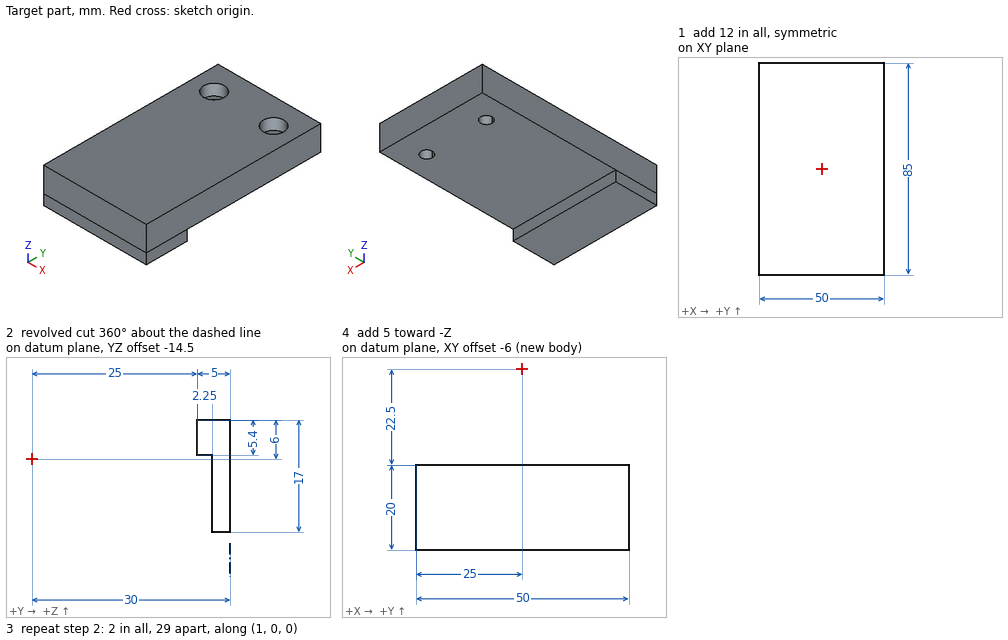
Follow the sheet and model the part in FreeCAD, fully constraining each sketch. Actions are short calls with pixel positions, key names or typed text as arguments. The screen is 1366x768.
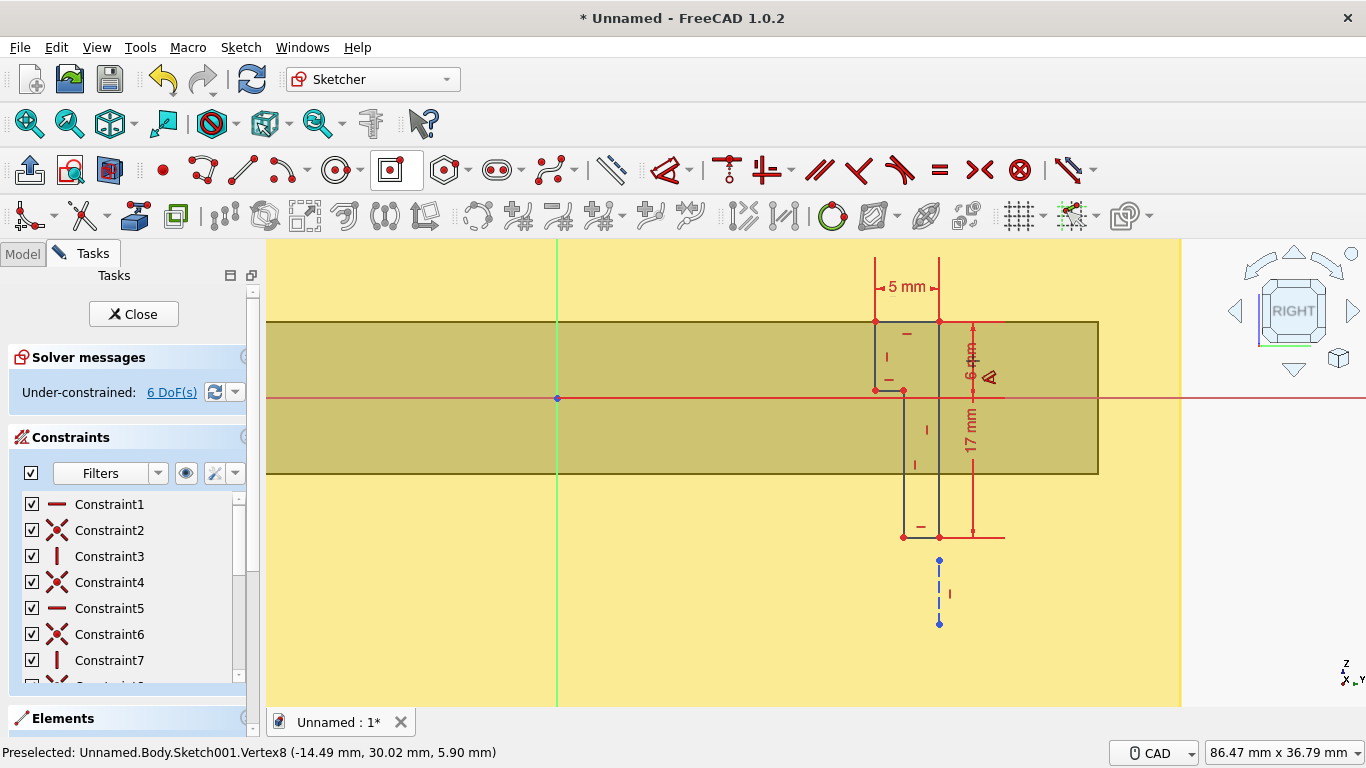
click(875, 342)
click(909, 340)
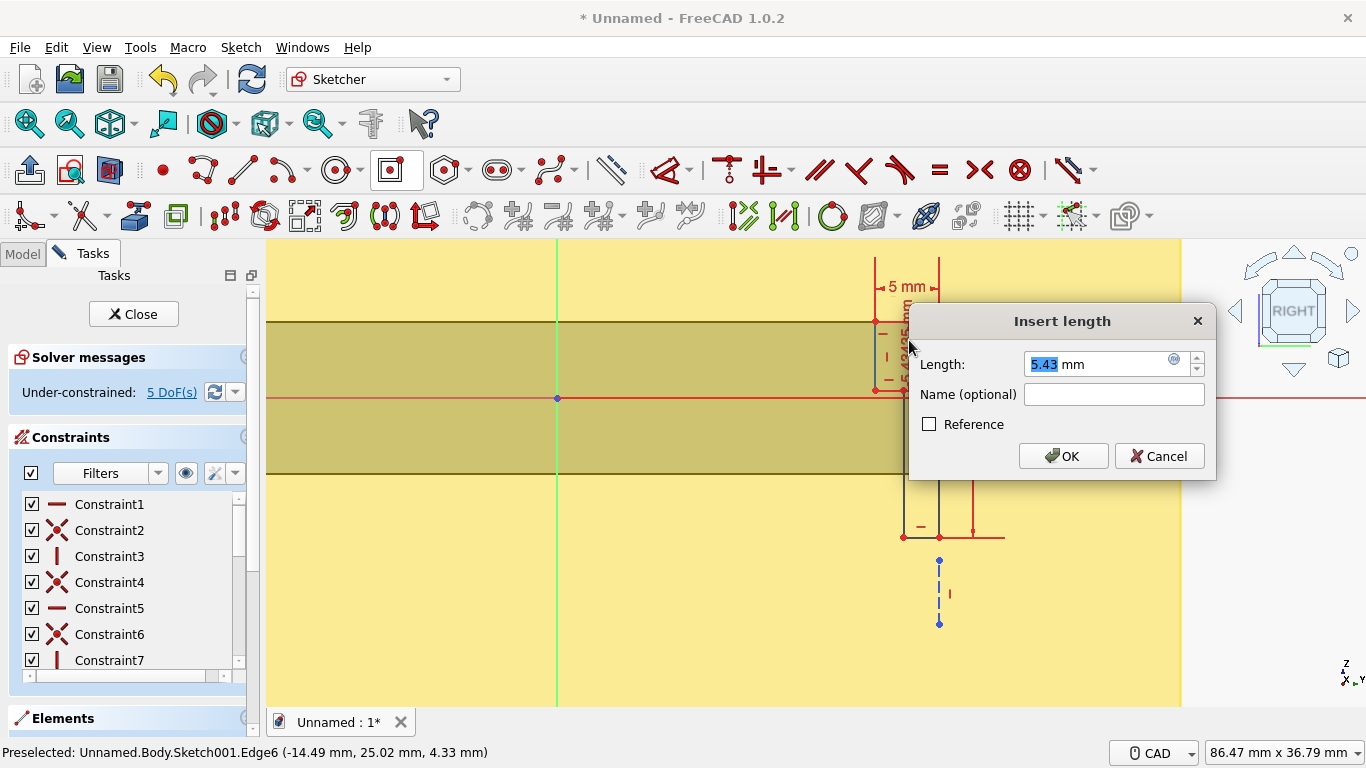
text(5.4)
key(Return)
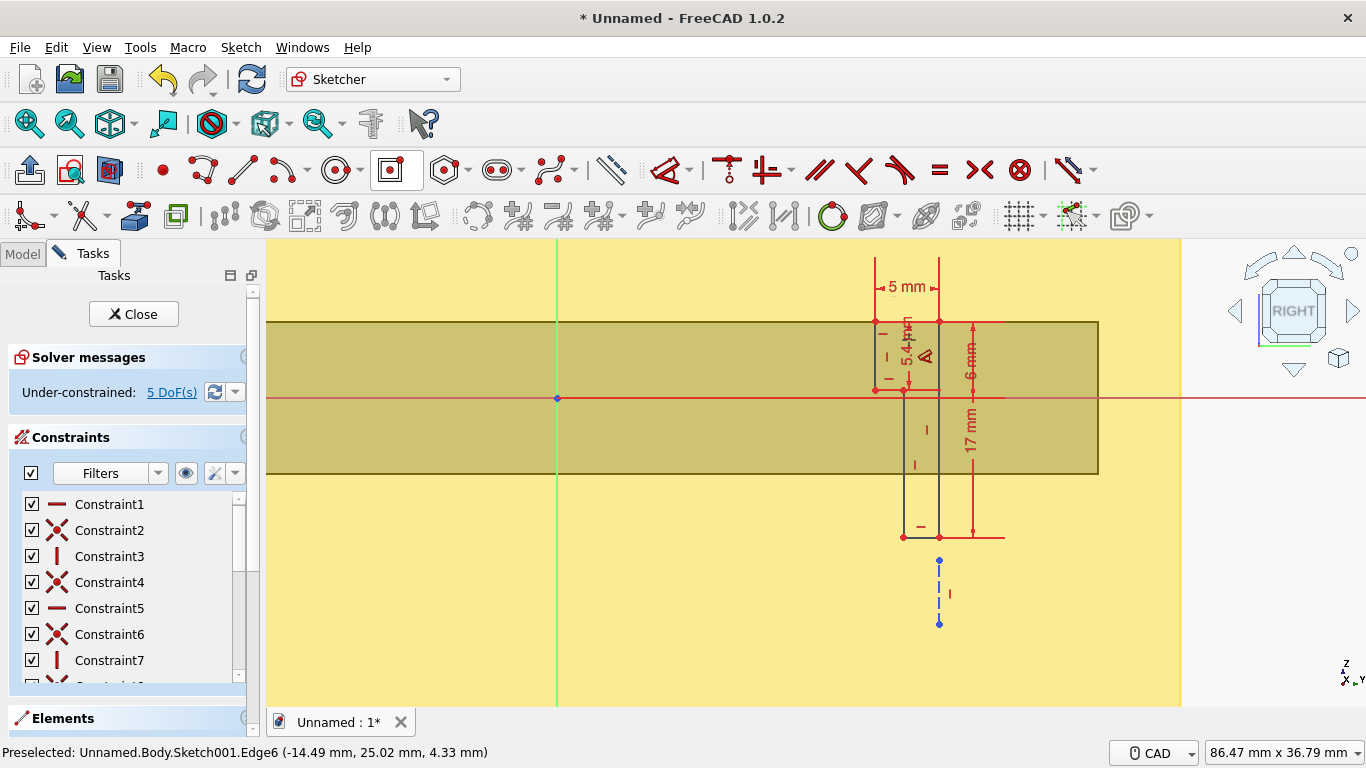
click(875, 390)
click(716, 356)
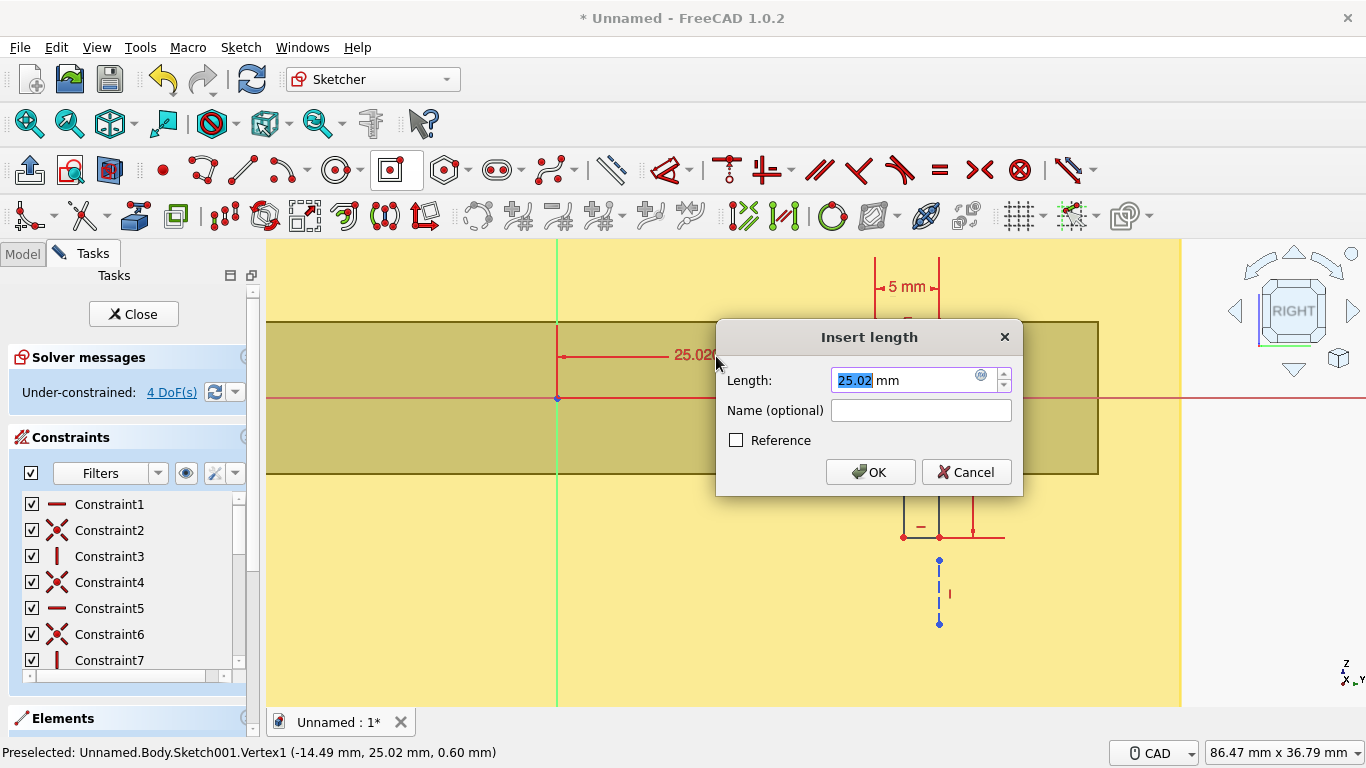
text(25)
key(Return)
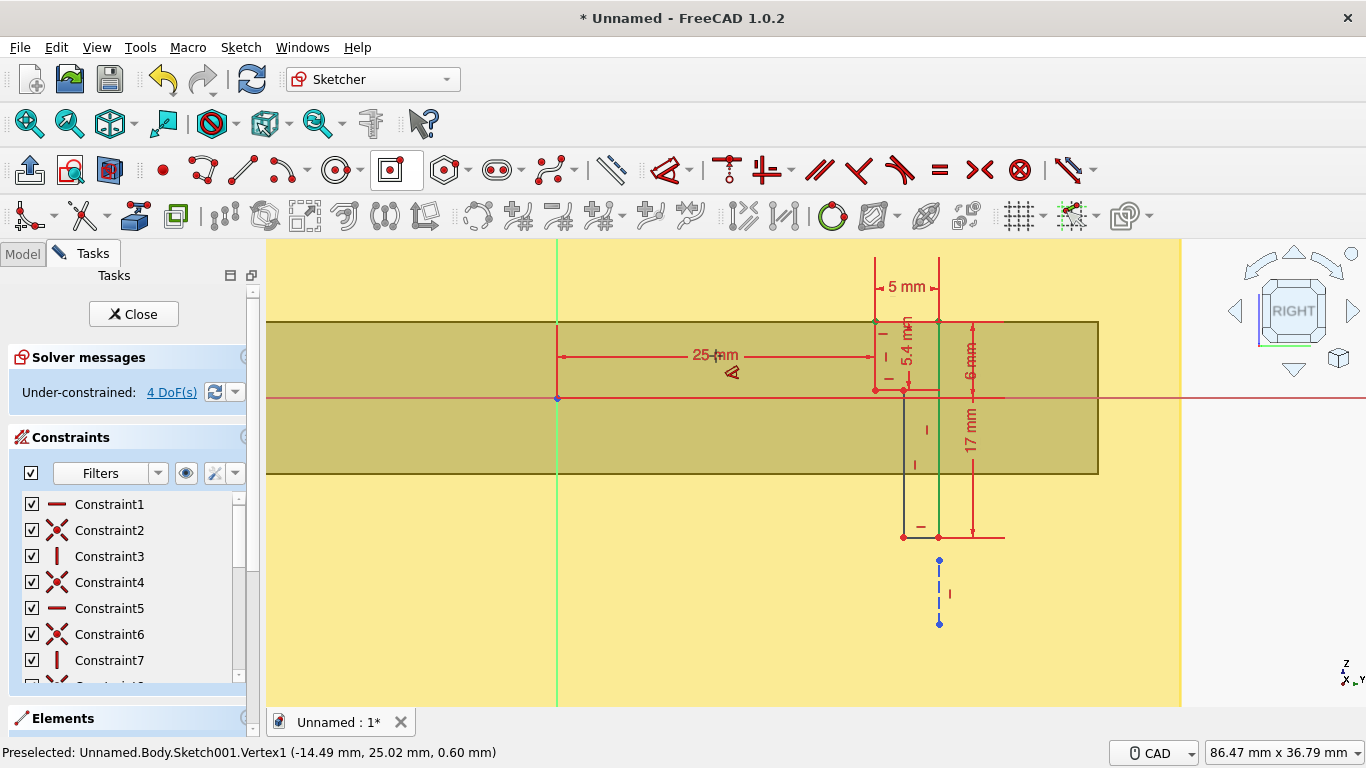
click(939, 561)
click(748, 595)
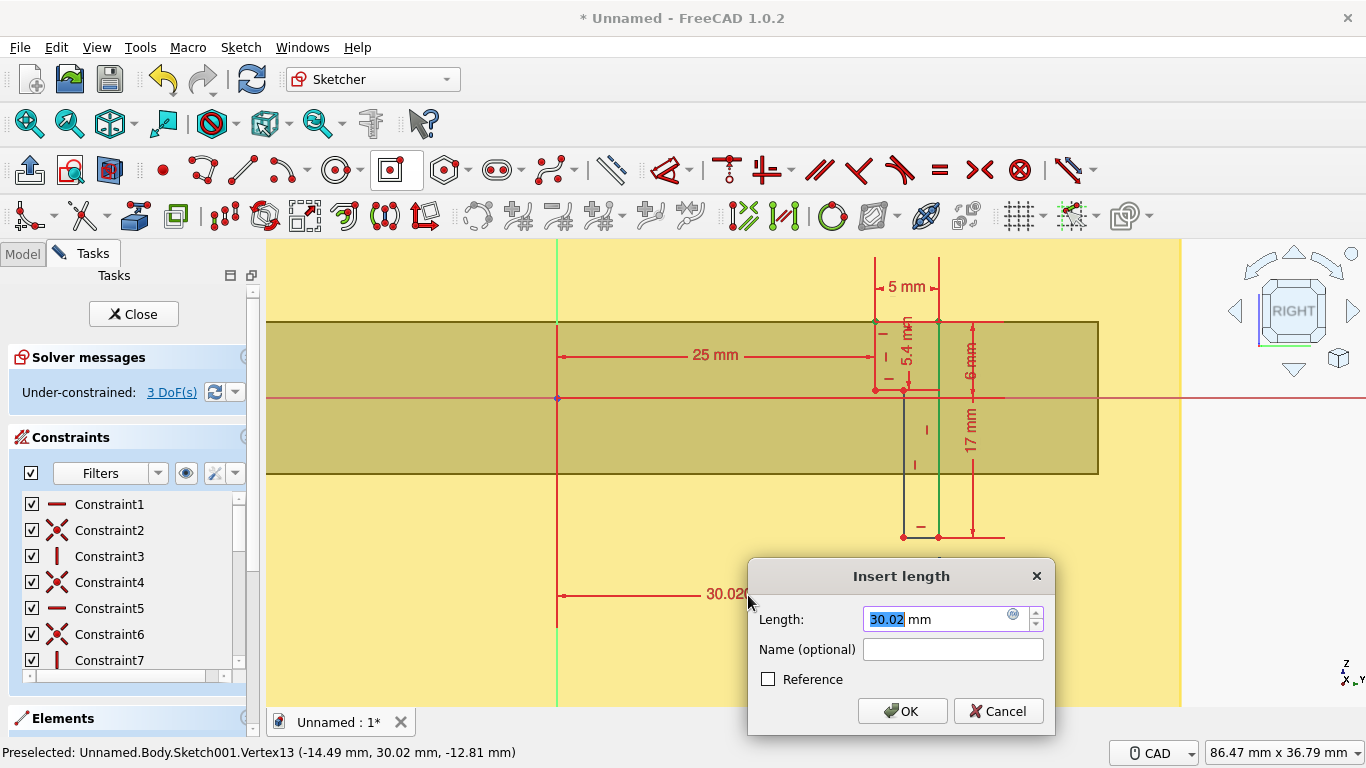
text(30)
key(Return)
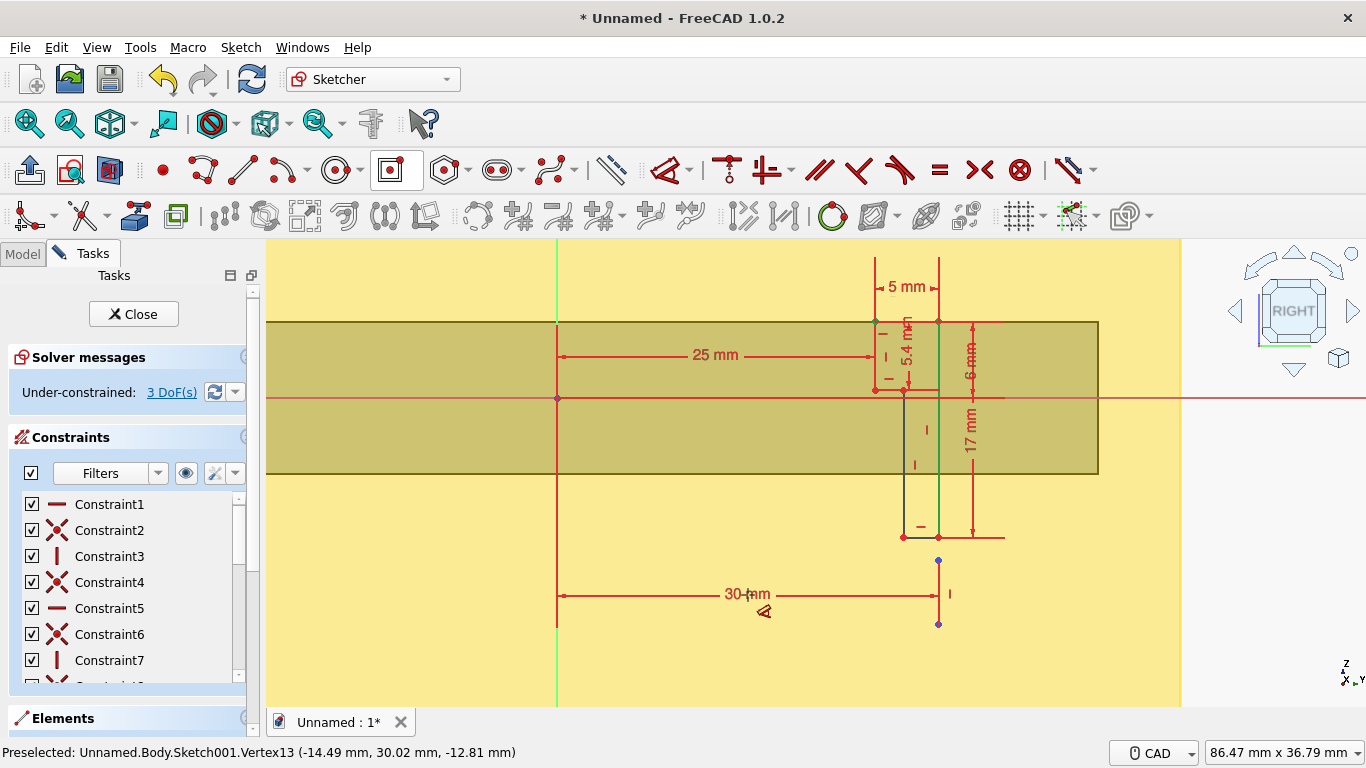
scroll(884, 390, up, 3)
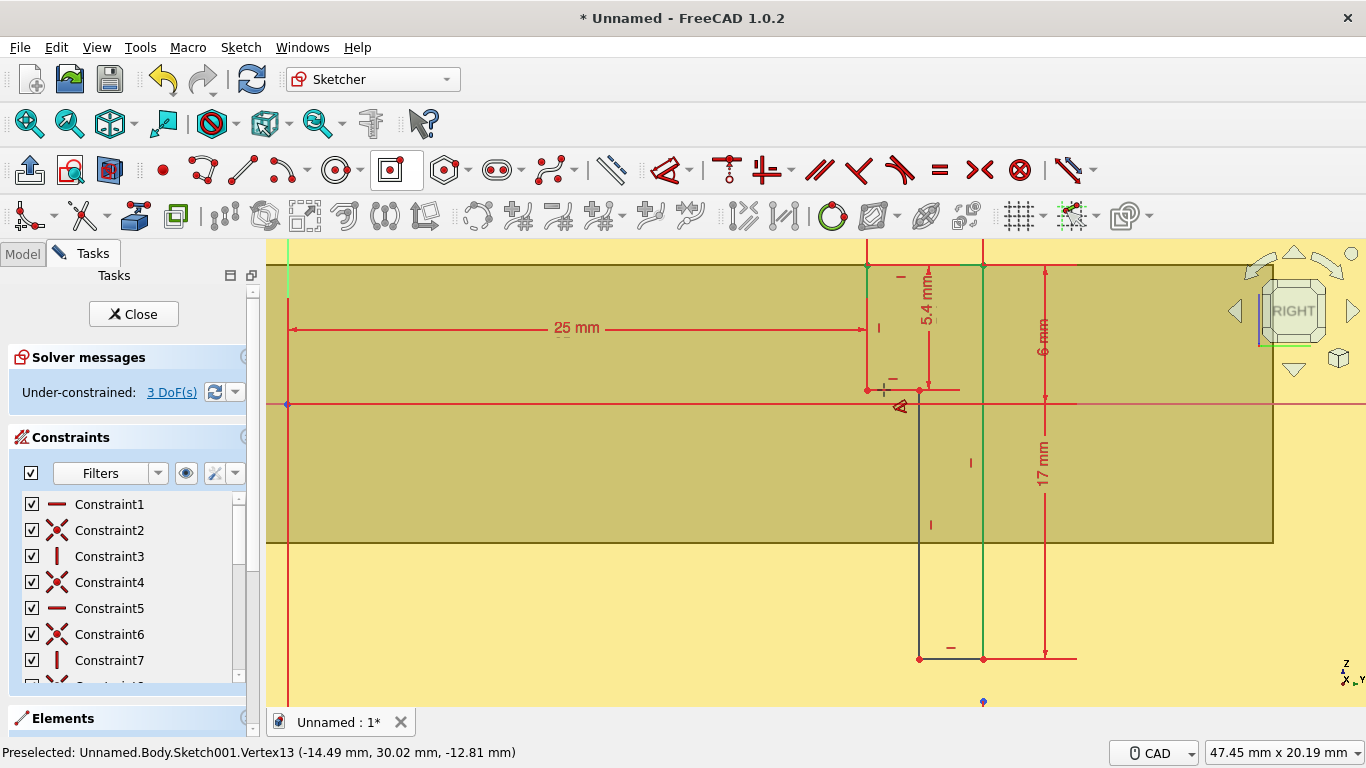
click(883, 390)
click(893, 356)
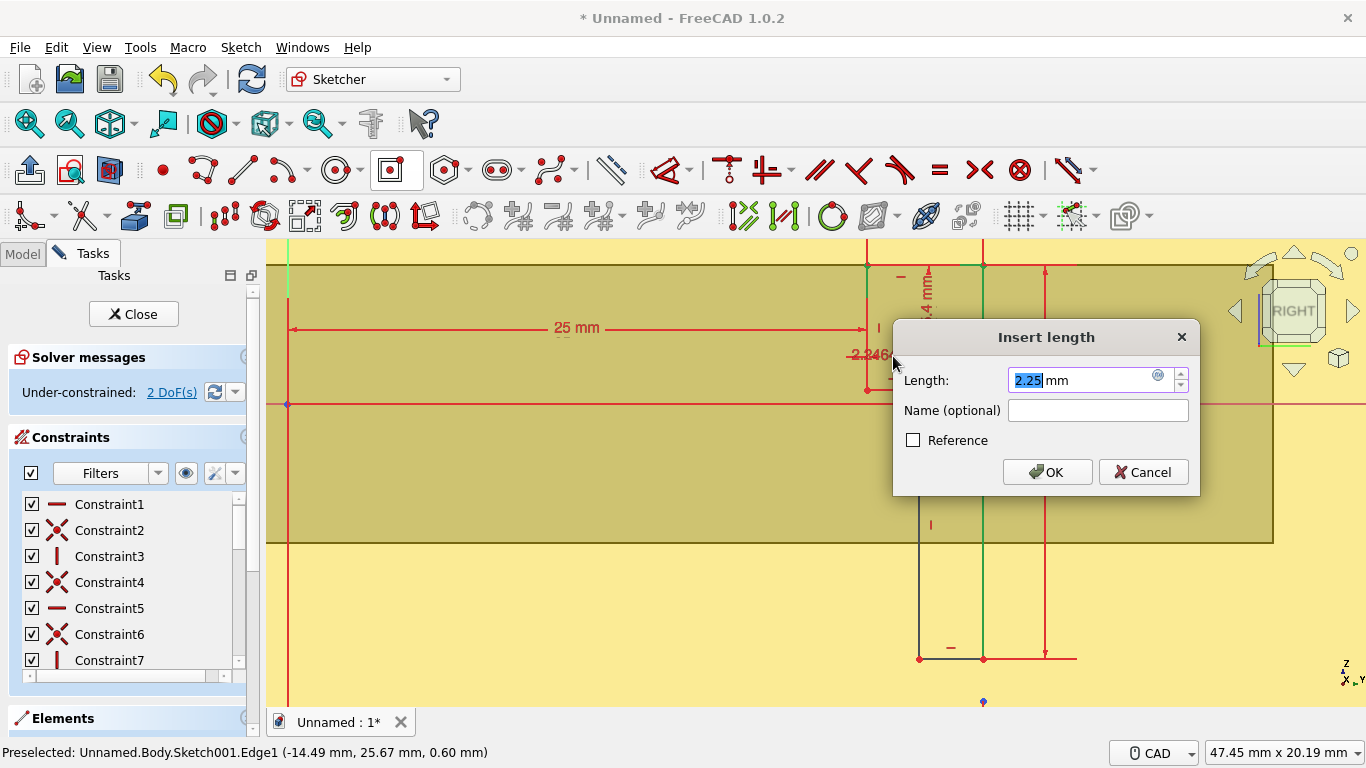
text(2.25)
key(Return)
key(Escape)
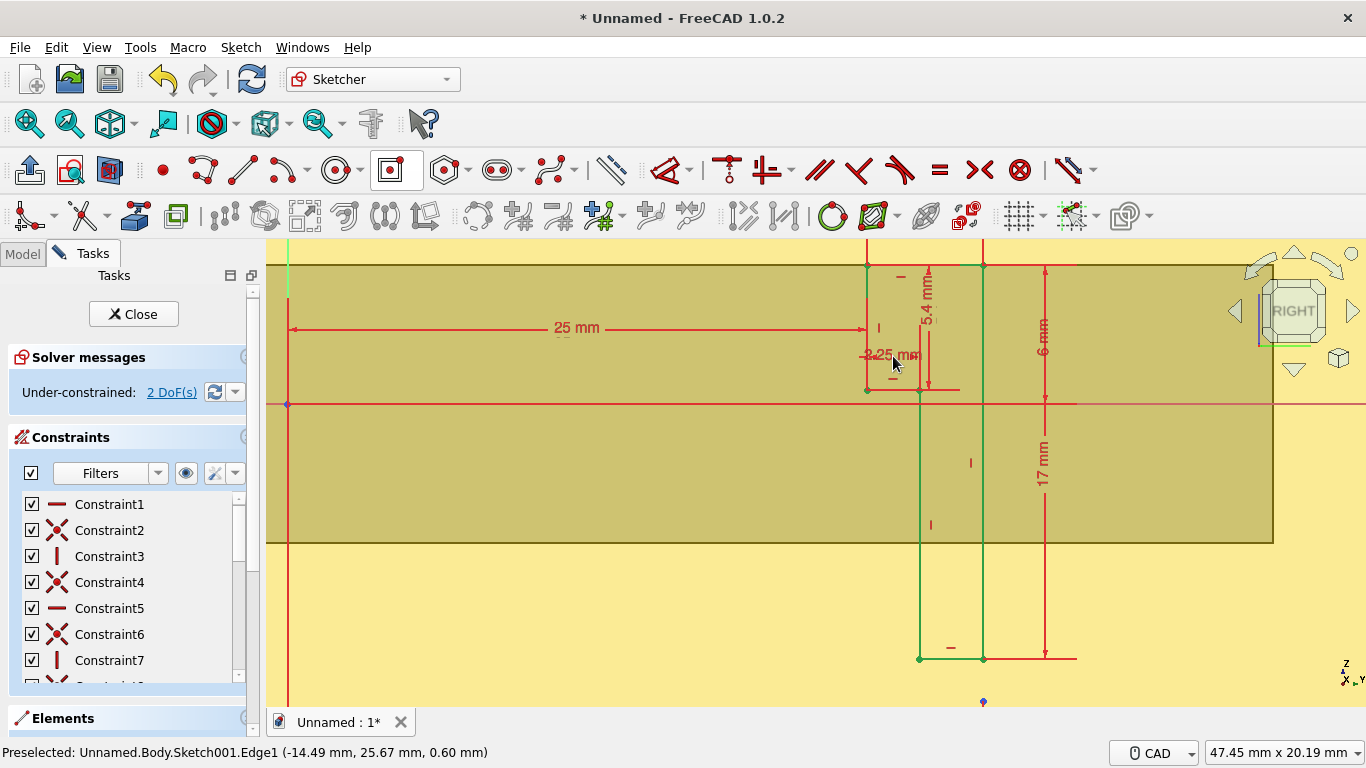
click(134, 314)